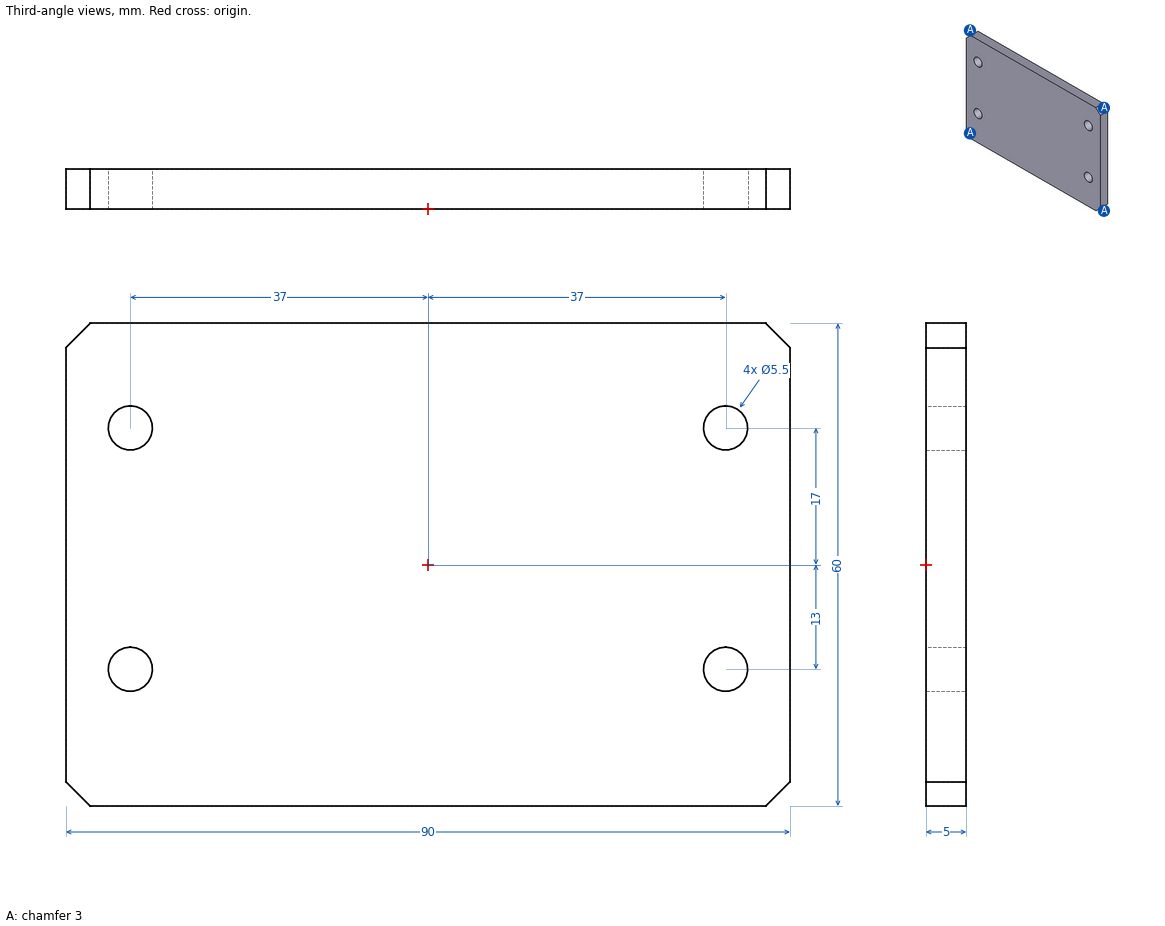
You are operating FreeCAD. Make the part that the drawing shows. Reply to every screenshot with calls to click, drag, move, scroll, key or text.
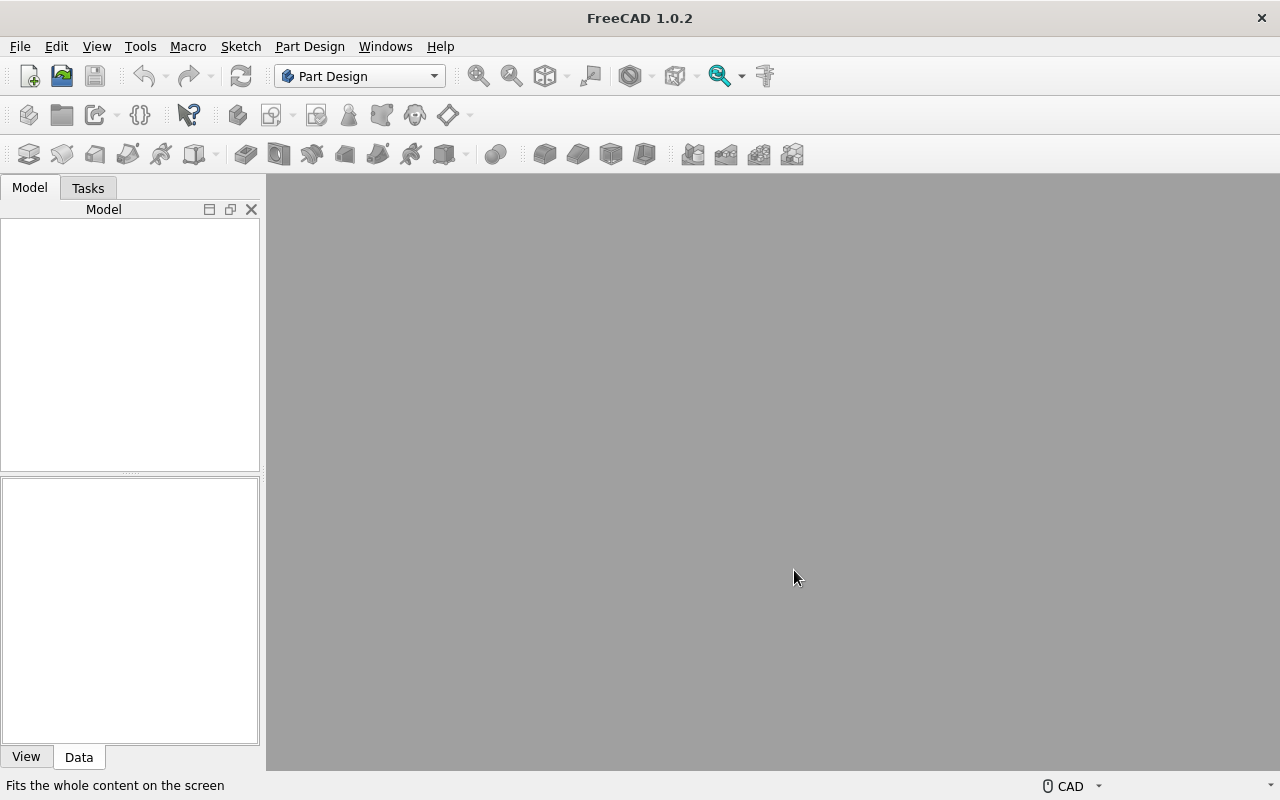
click(29, 76)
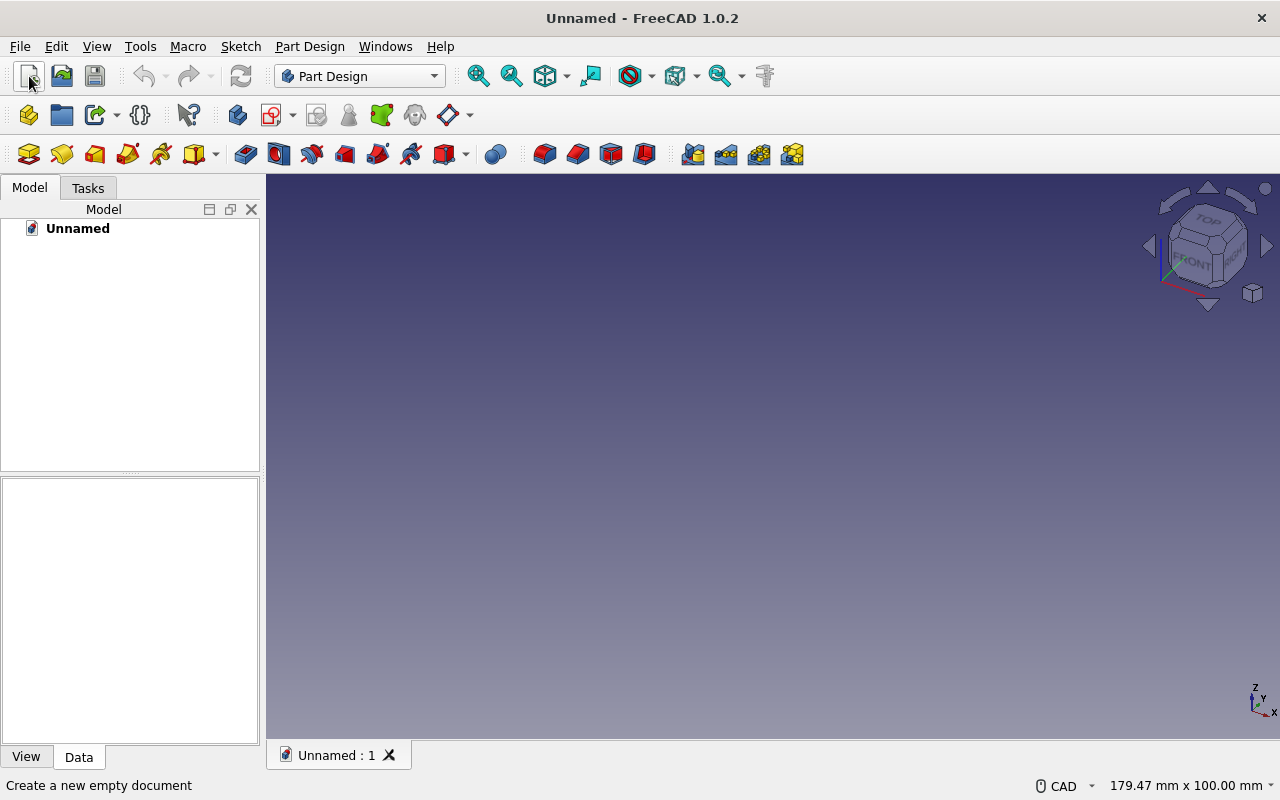
click(270, 116)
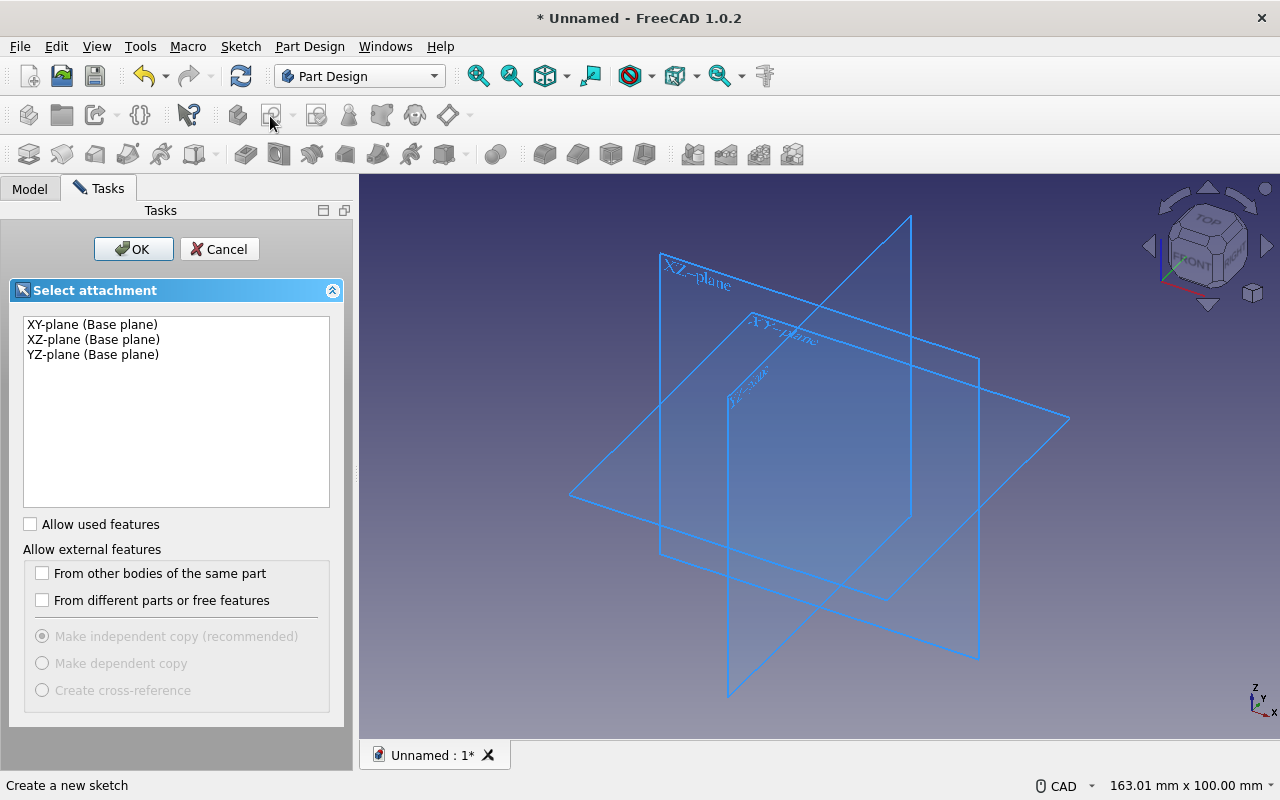
click(84, 340)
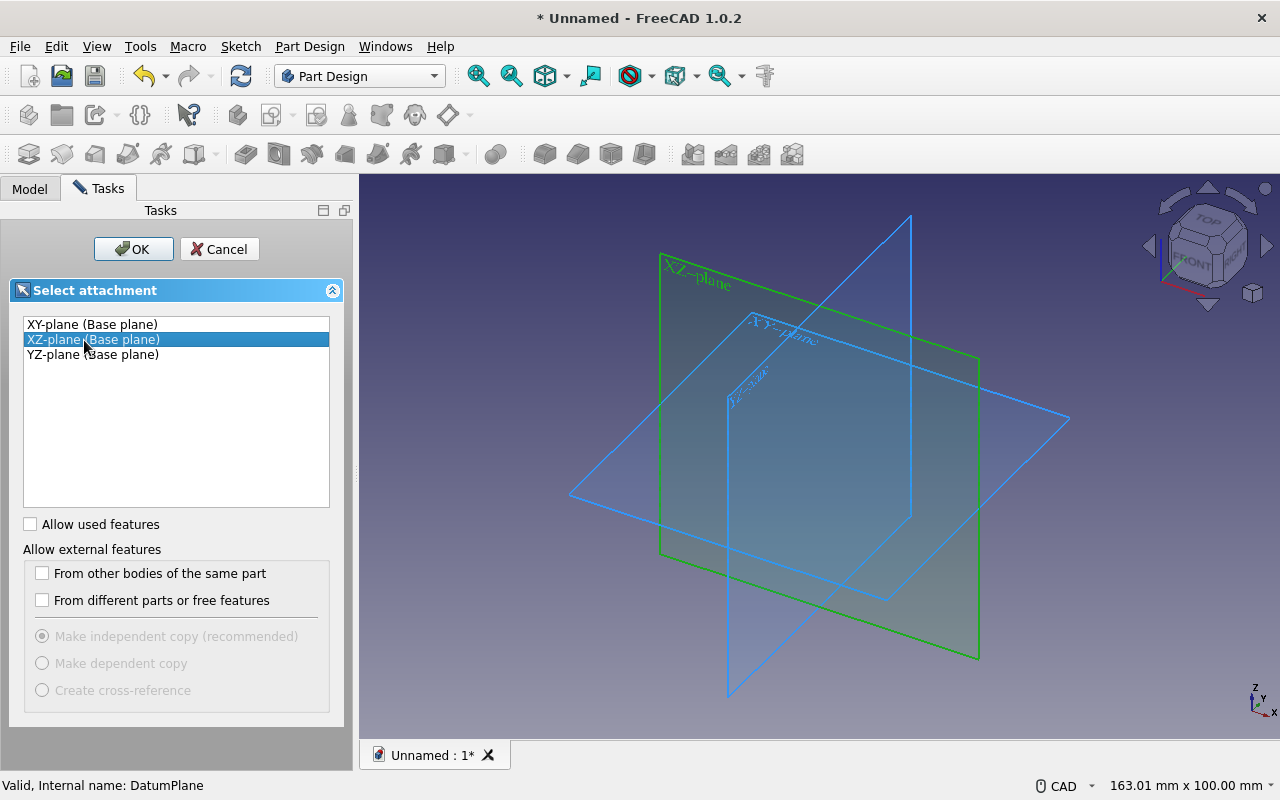
click(134, 249)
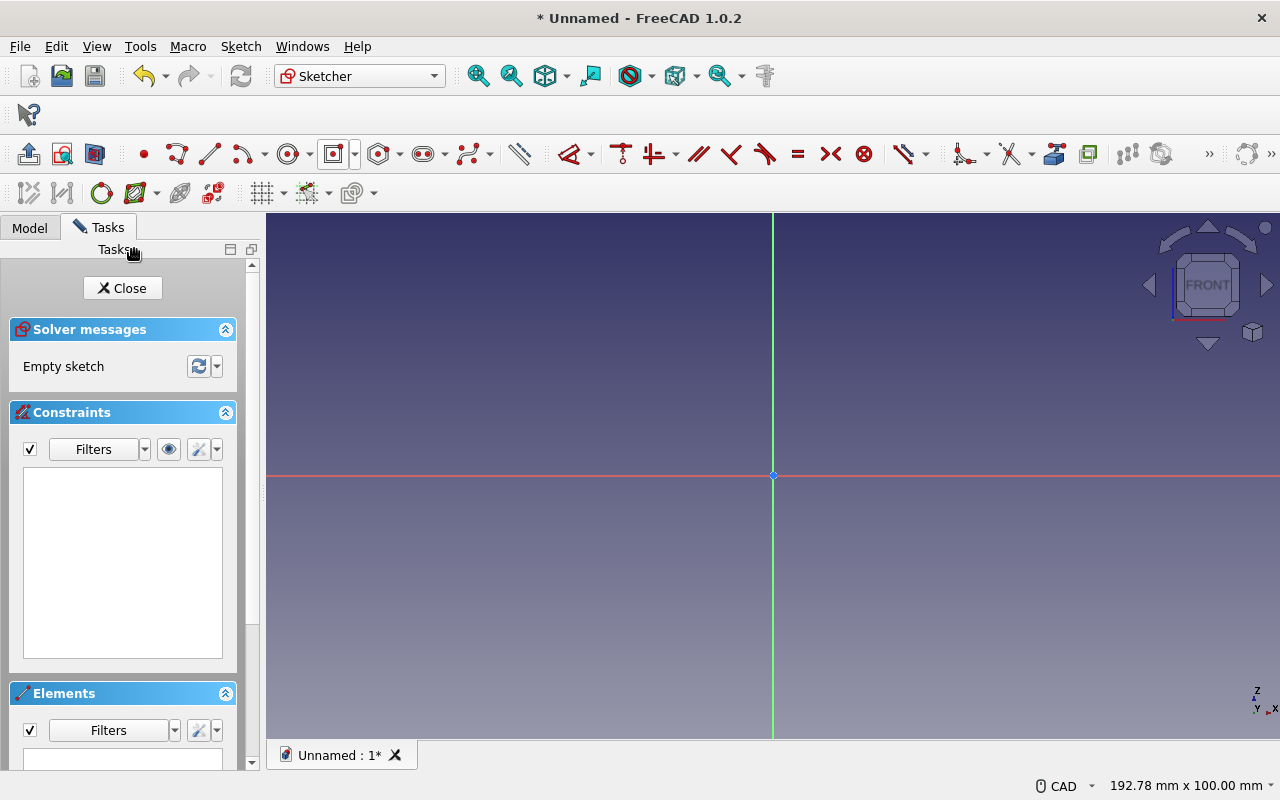
click(332, 154)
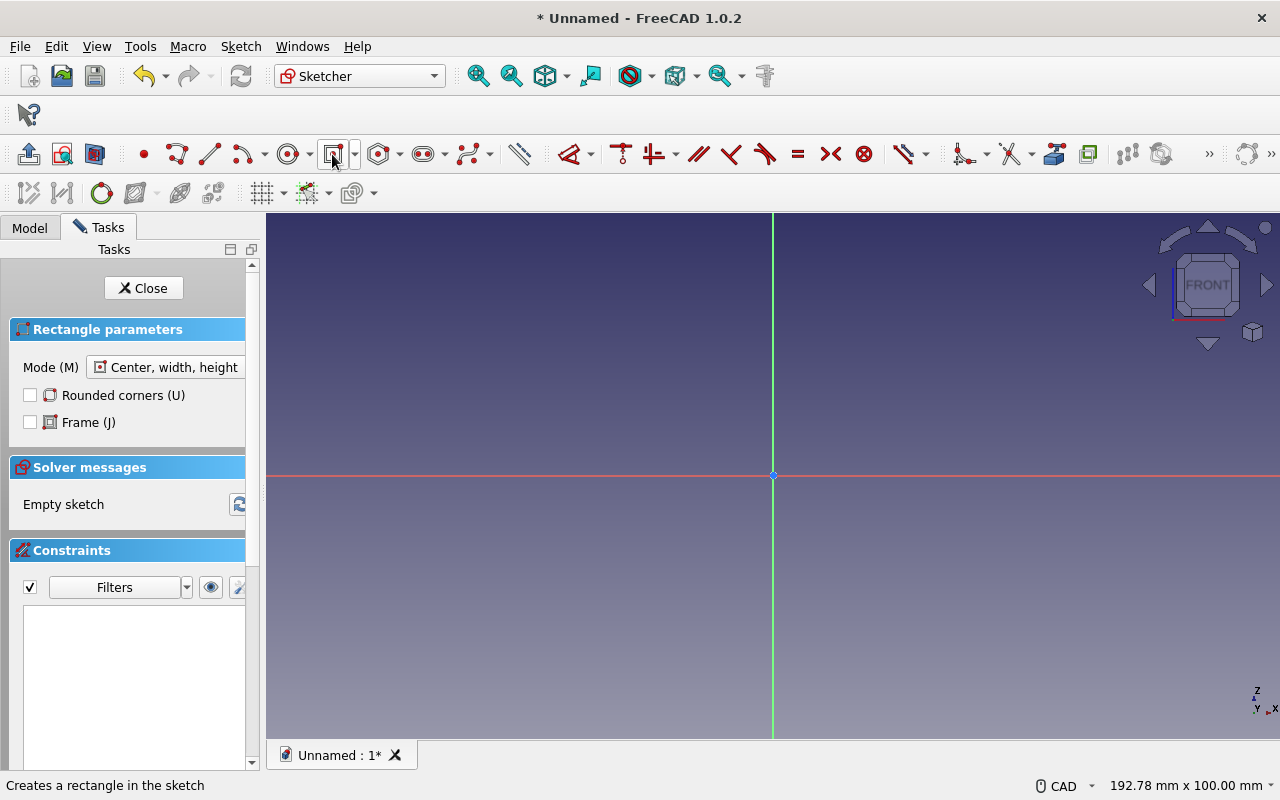
click(773, 476)
click(1010, 318)
key(Escape)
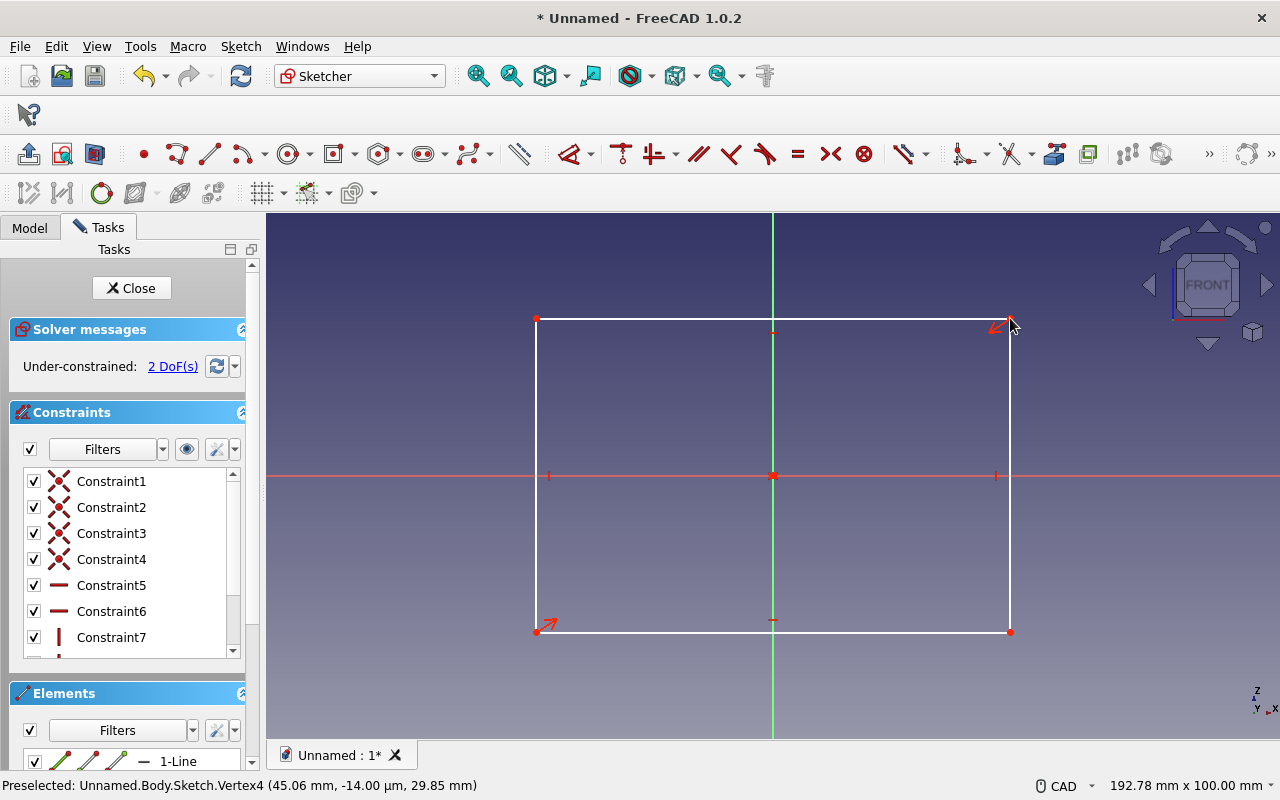
click(568, 154)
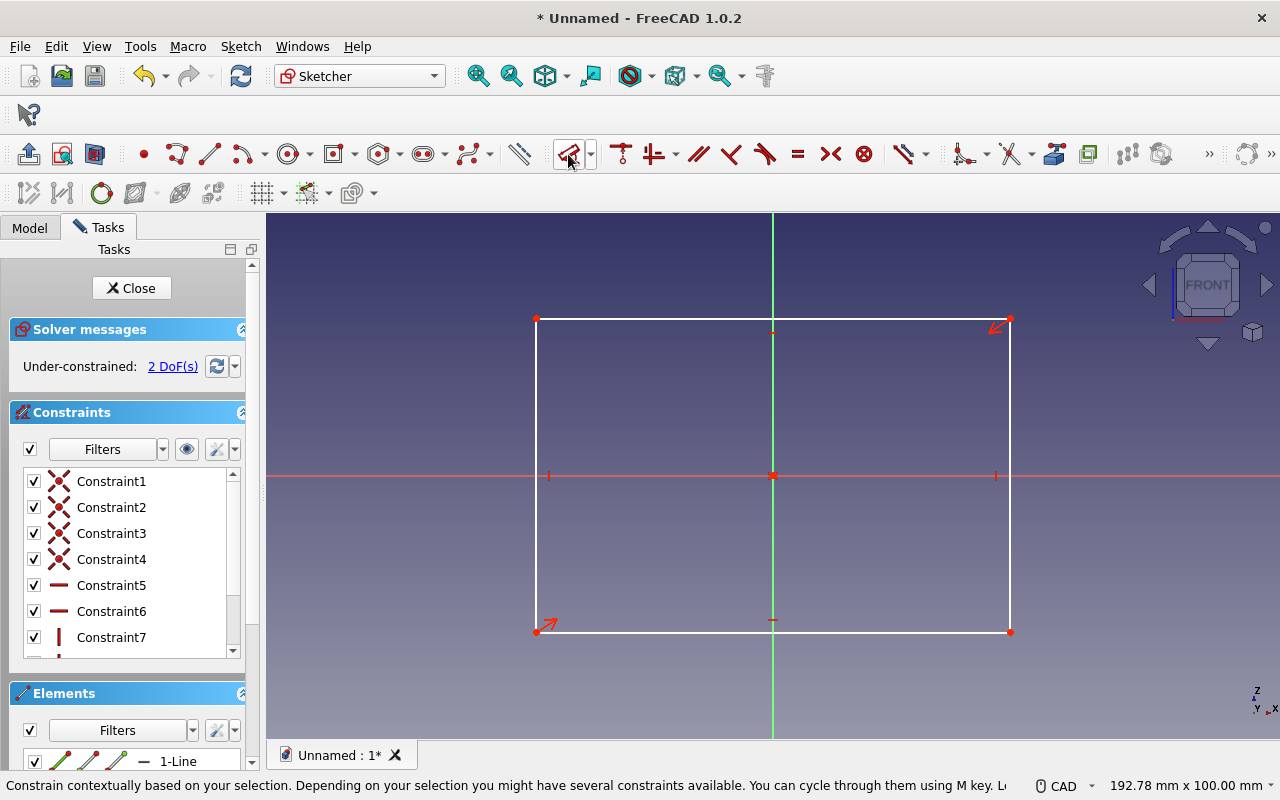
click(678, 633)
click(664, 667)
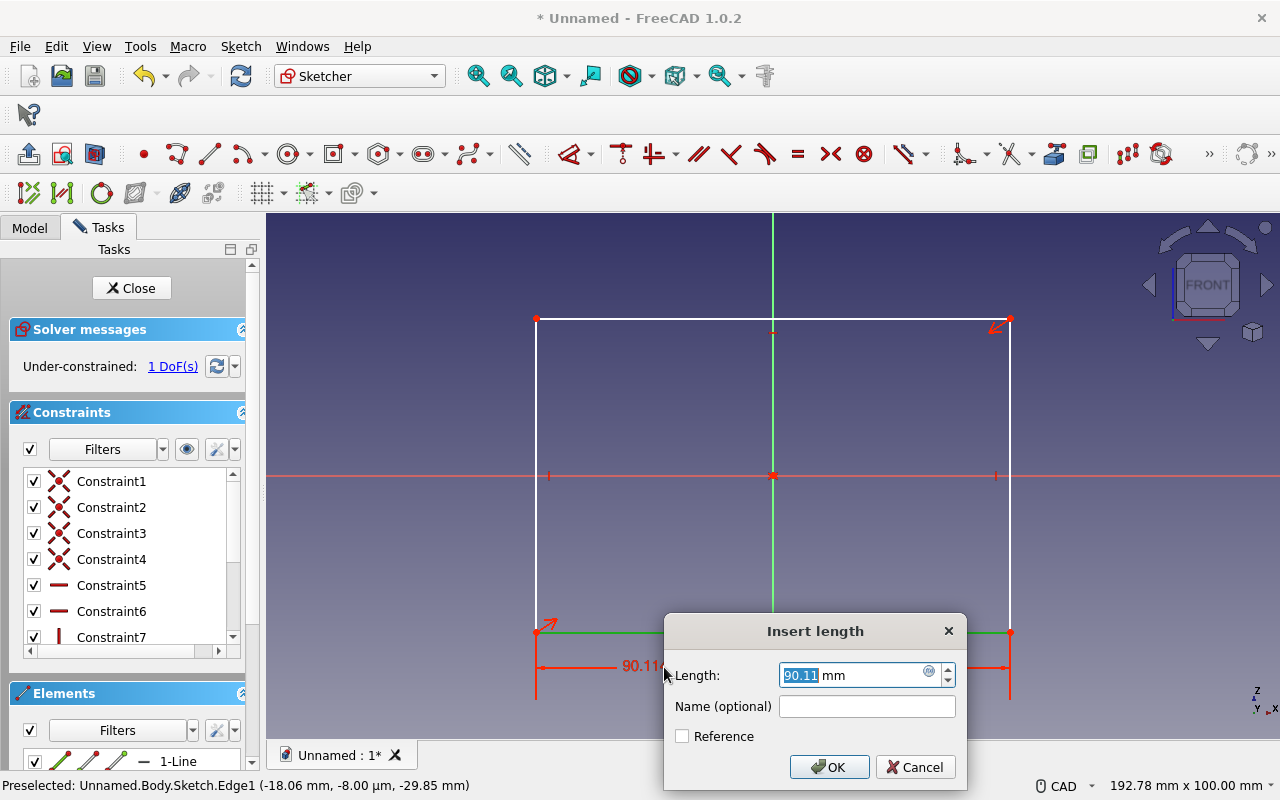
text(90)
key(Return)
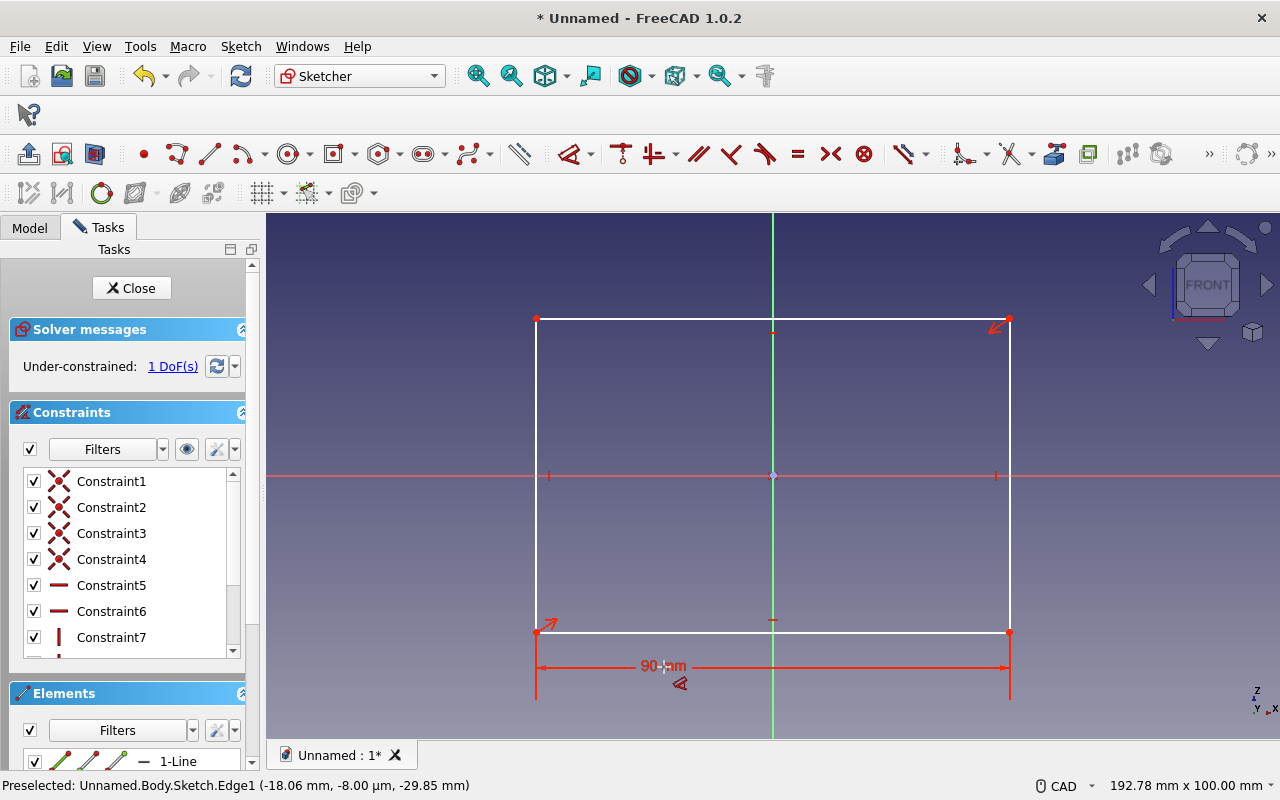
click(1010, 539)
click(1044, 404)